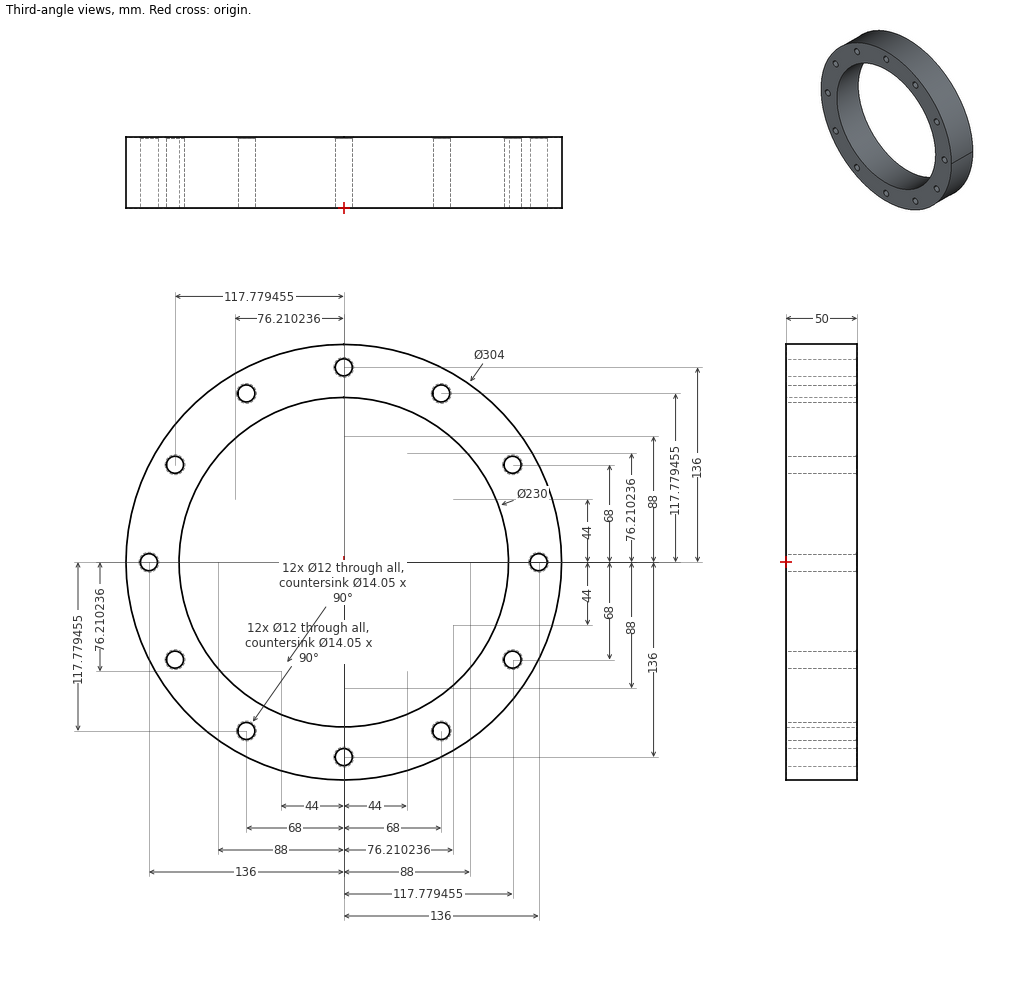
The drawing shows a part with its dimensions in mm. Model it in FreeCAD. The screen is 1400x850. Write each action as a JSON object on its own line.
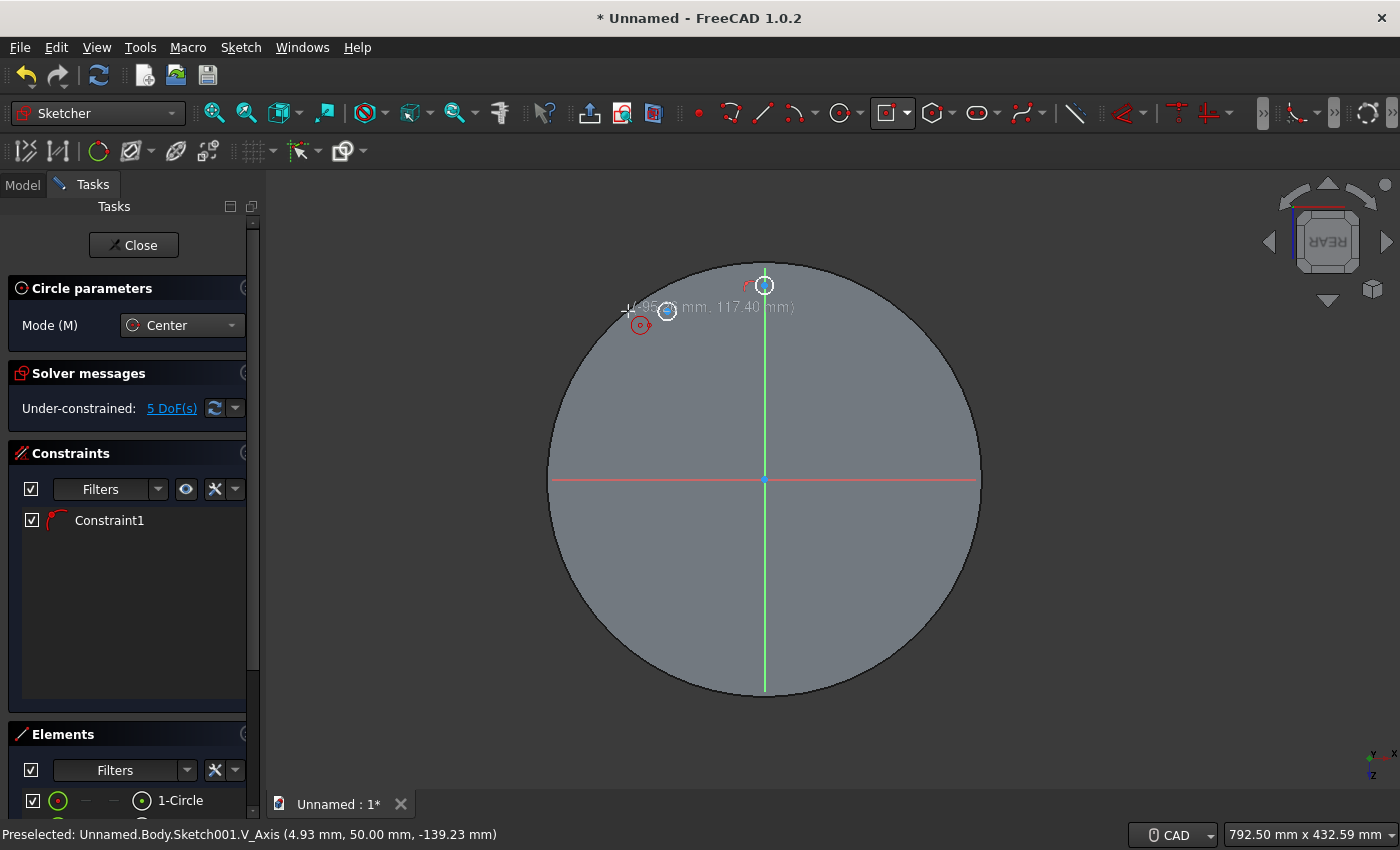
{"action": "scroll", "coordinate": [862, 311], "scroll_direction": "up", "scroll_amount": 5}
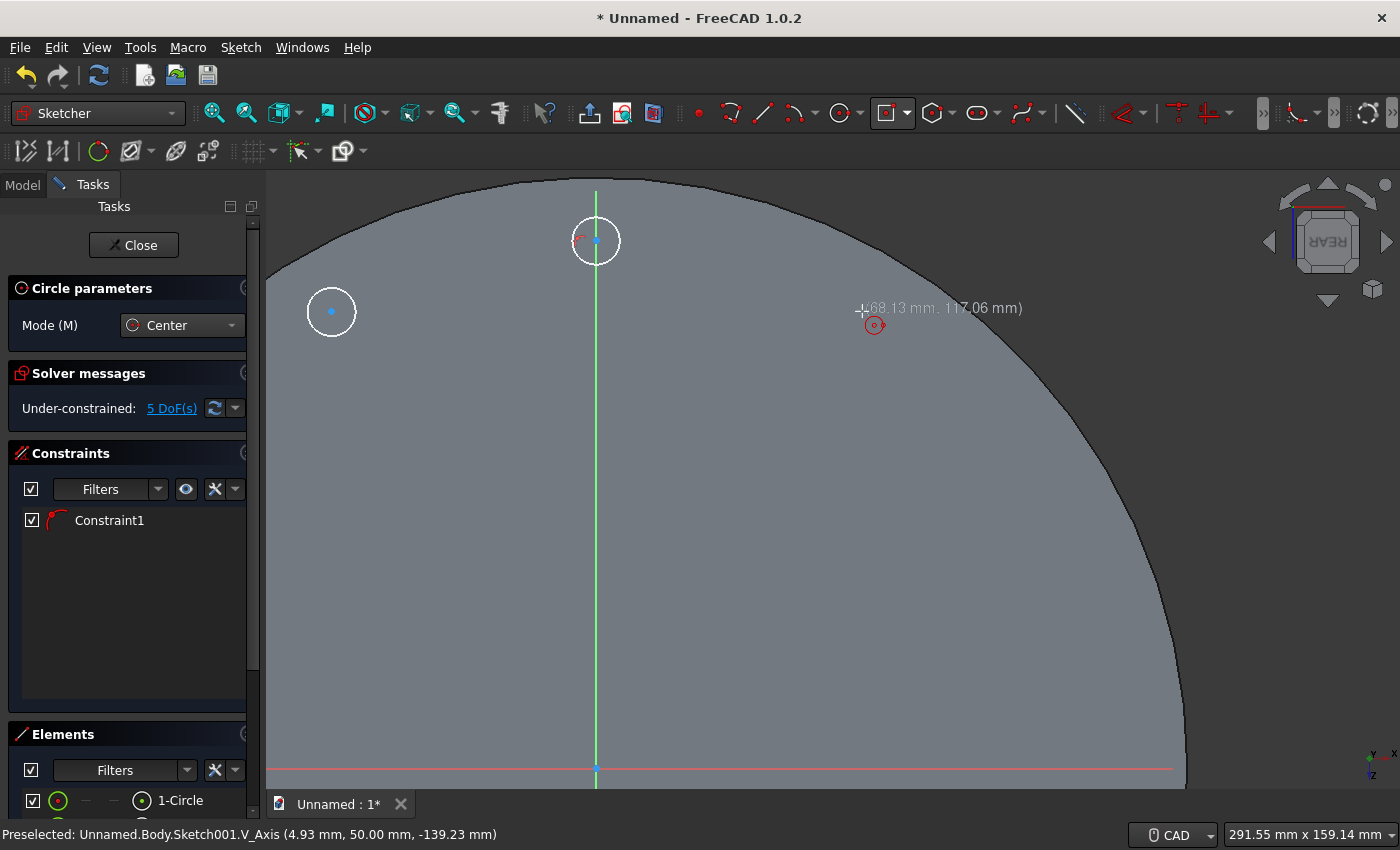
{"action": "left_click", "coordinate": [861, 311]}
{"action": "left_click", "coordinate": [877, 294]}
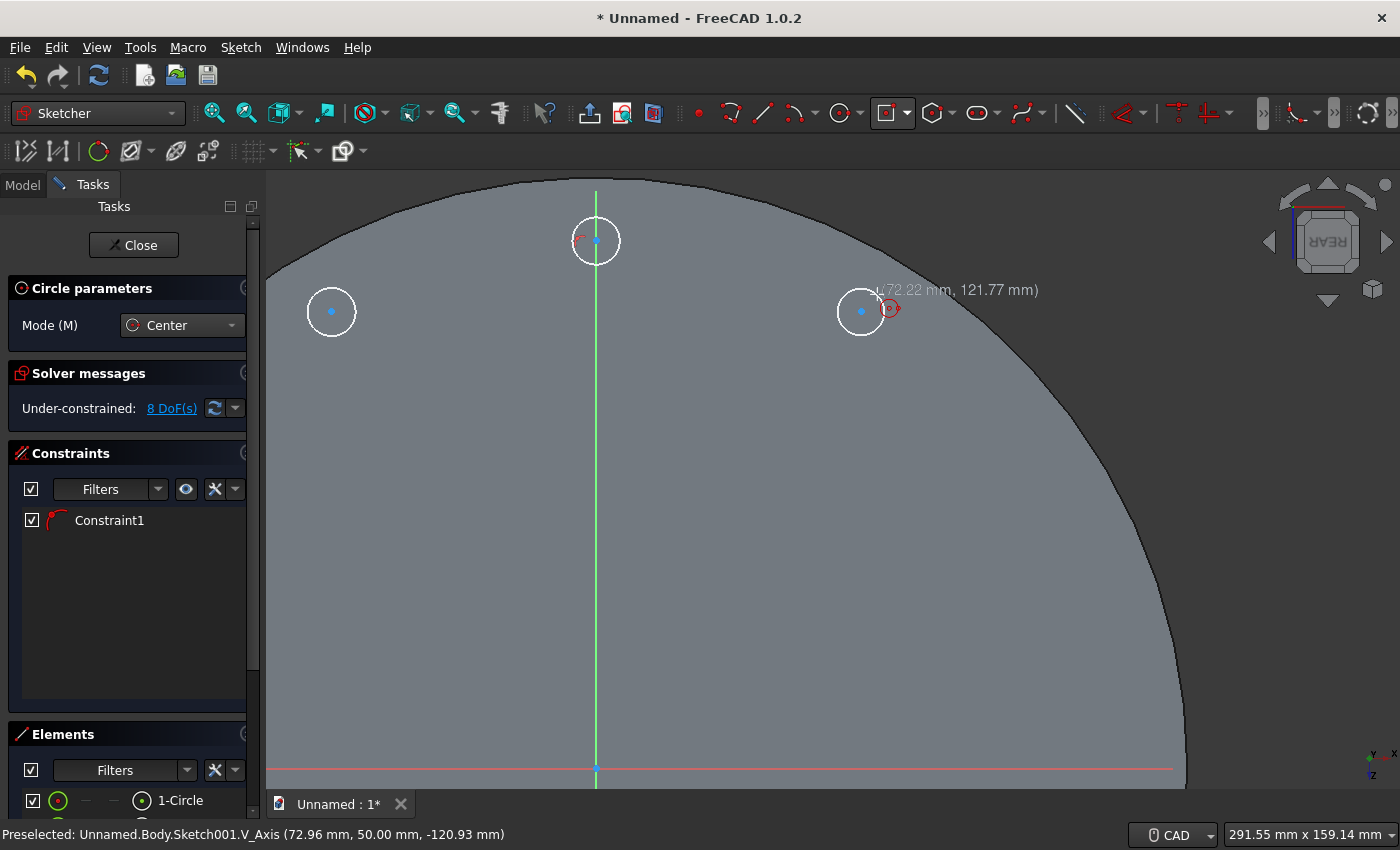
{"action": "left_click", "coordinate": [1054, 504]}
{"action": "left_click", "coordinate": [1071, 488]}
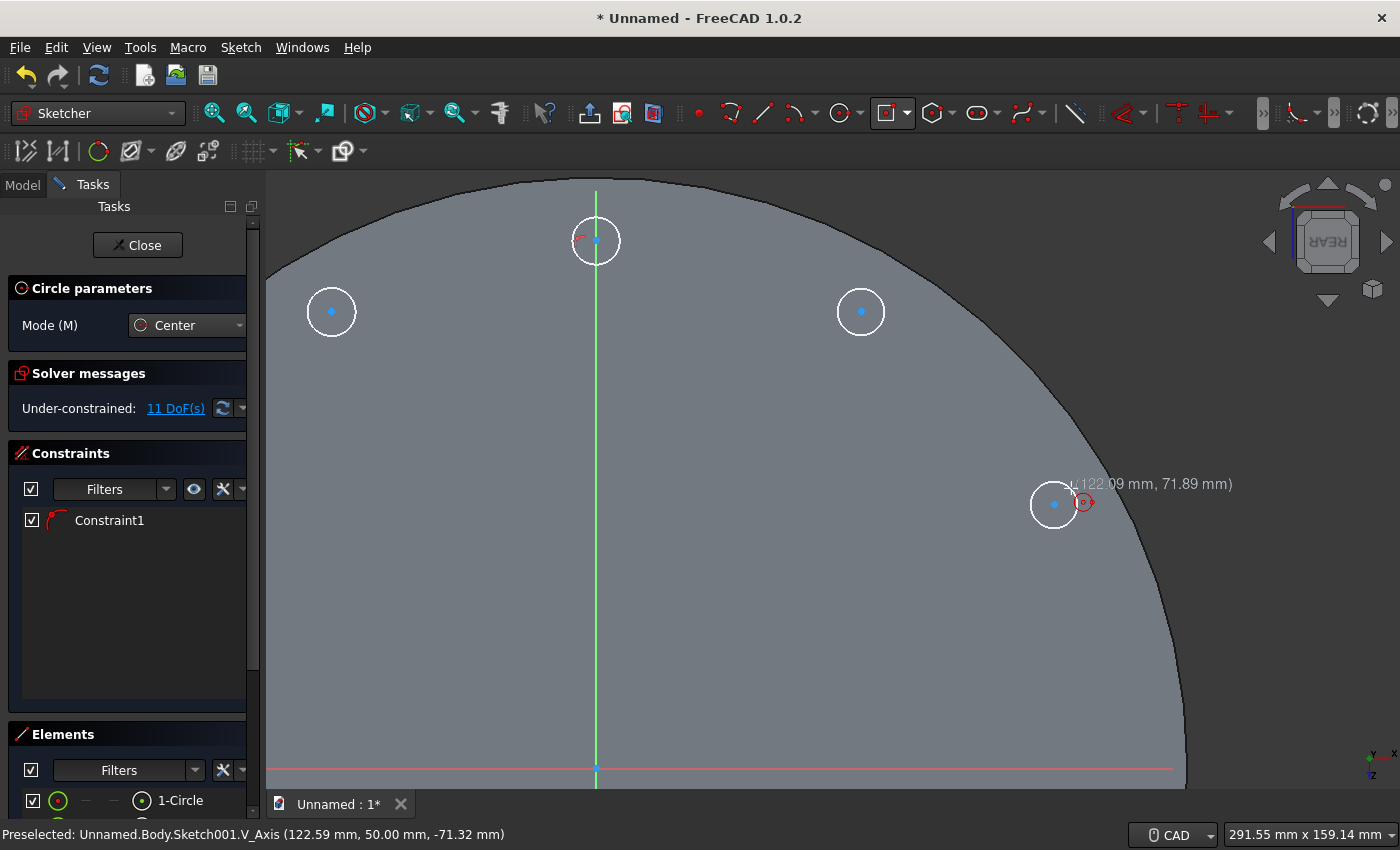
{"action": "scroll", "coordinate": [862, 311], "scroll_direction": "down", "scroll_amount": 5}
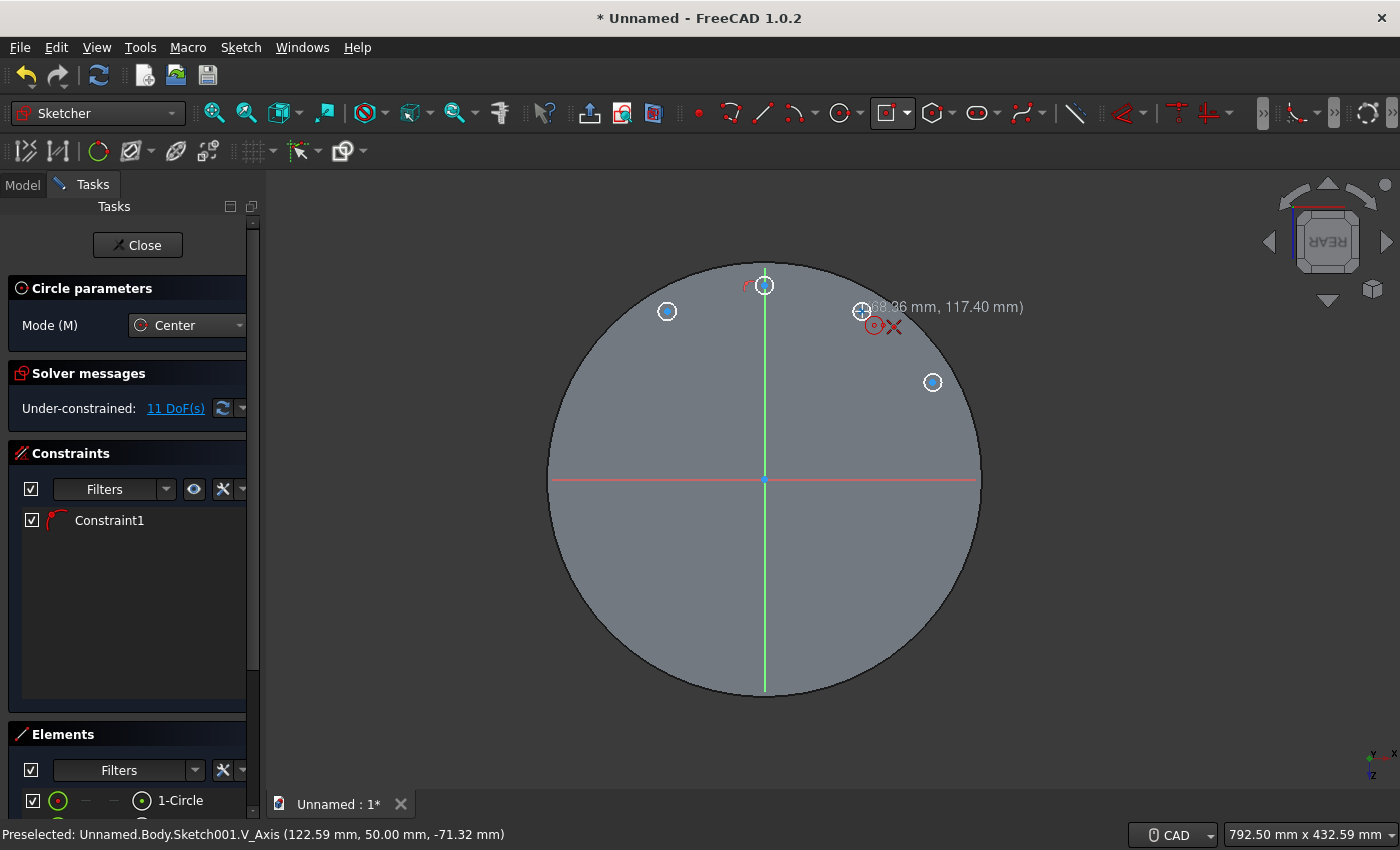
{"action": "scroll", "coordinate": [959, 480], "scroll_direction": "up", "scroll_amount": 5}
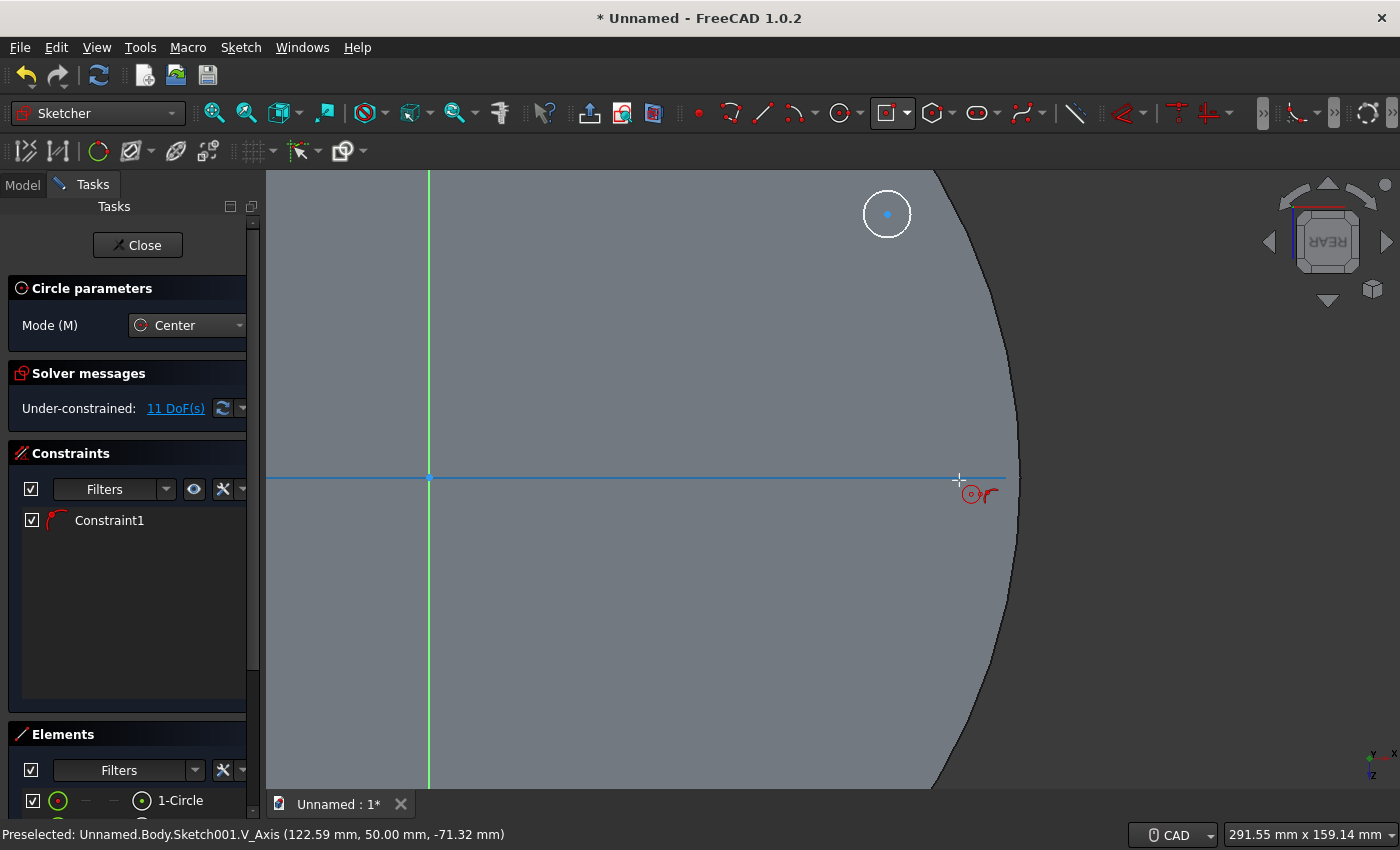
{"action": "left_click", "coordinate": [958, 478]}
{"action": "left_click", "coordinate": [975, 461]}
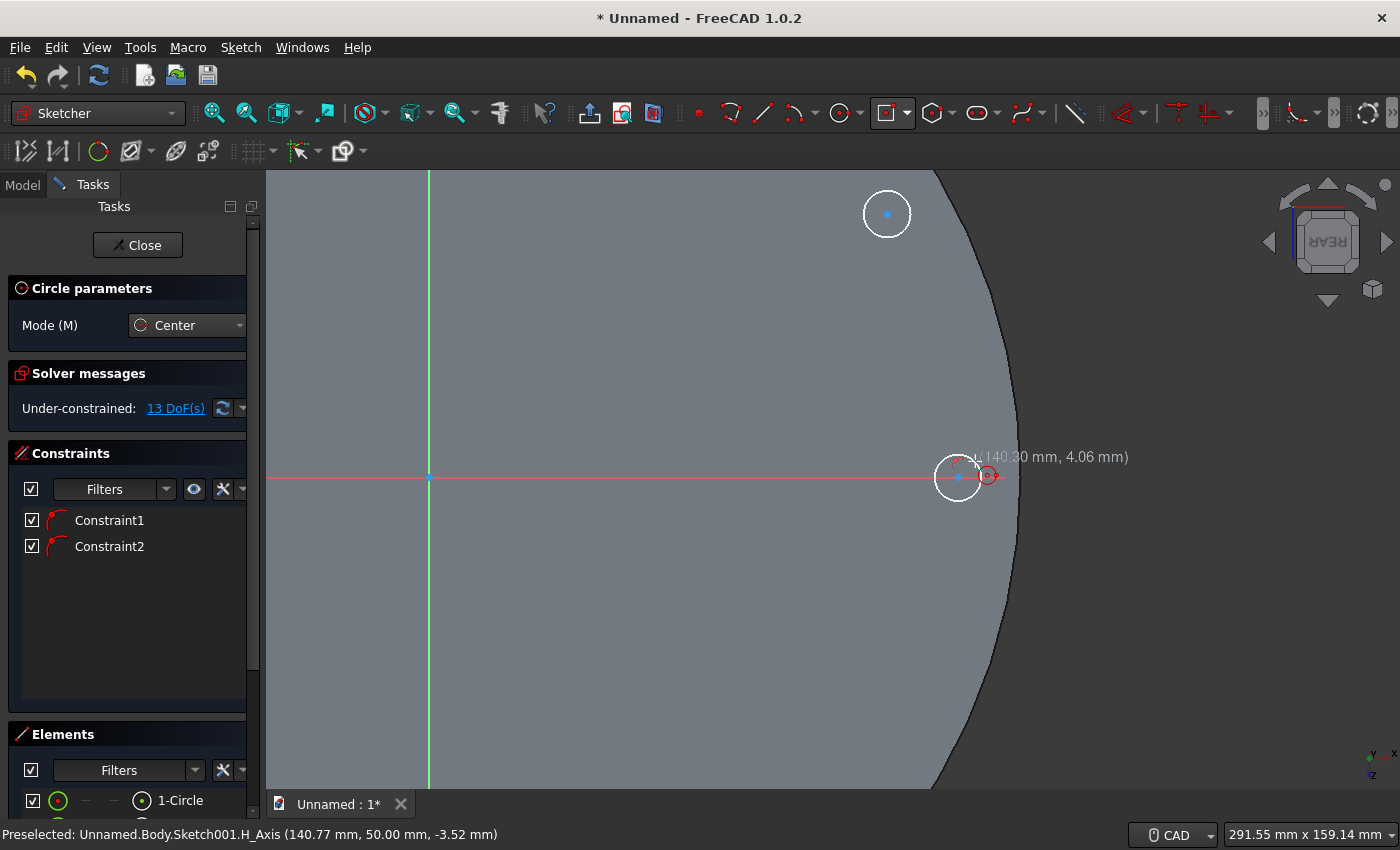
{"action": "left_click", "coordinate": [887, 742]}
{"action": "left_click", "coordinate": [904, 726]}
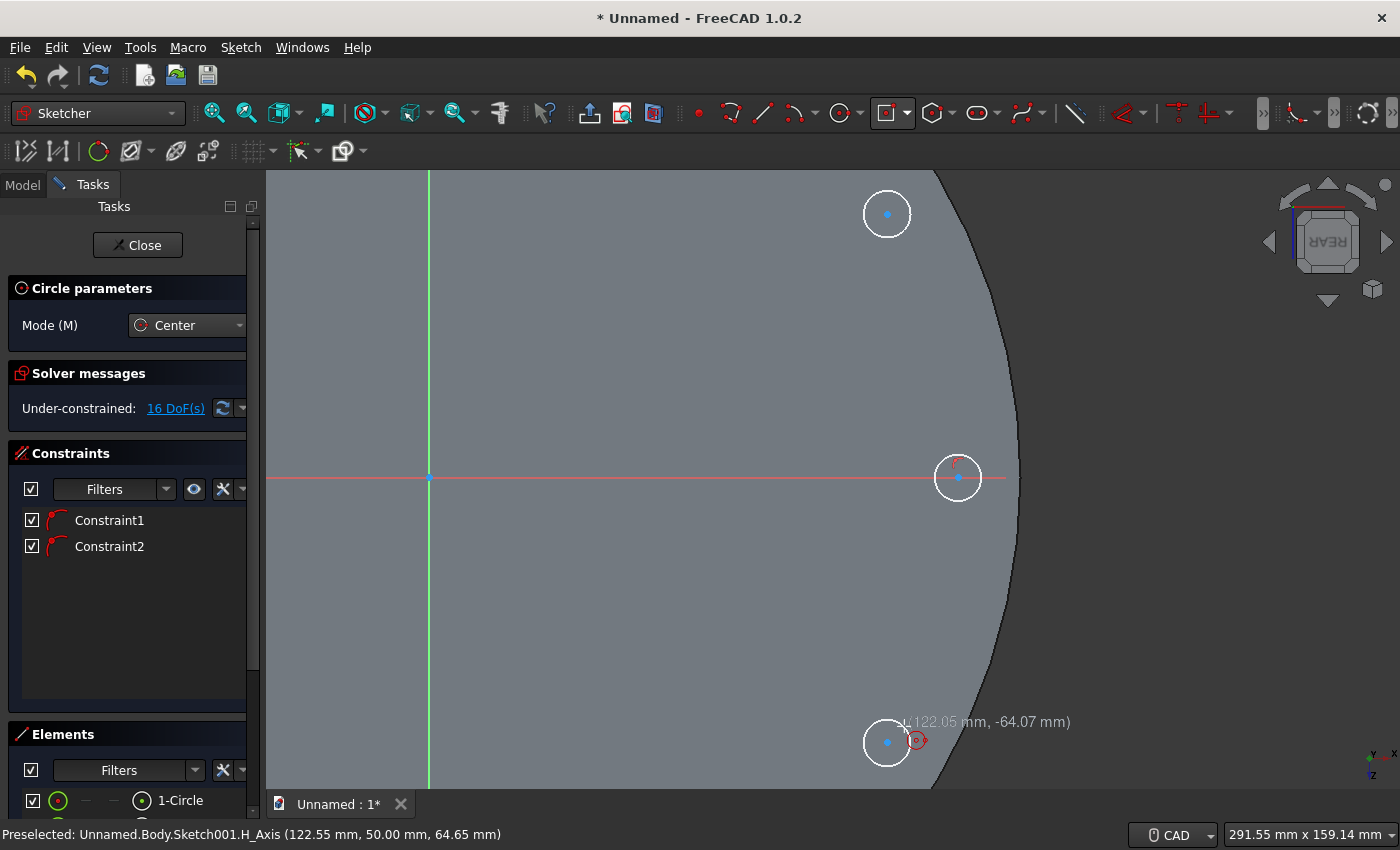
{"action": "scroll", "coordinate": [960, 481], "scroll_direction": "down", "scroll_amount": 5}